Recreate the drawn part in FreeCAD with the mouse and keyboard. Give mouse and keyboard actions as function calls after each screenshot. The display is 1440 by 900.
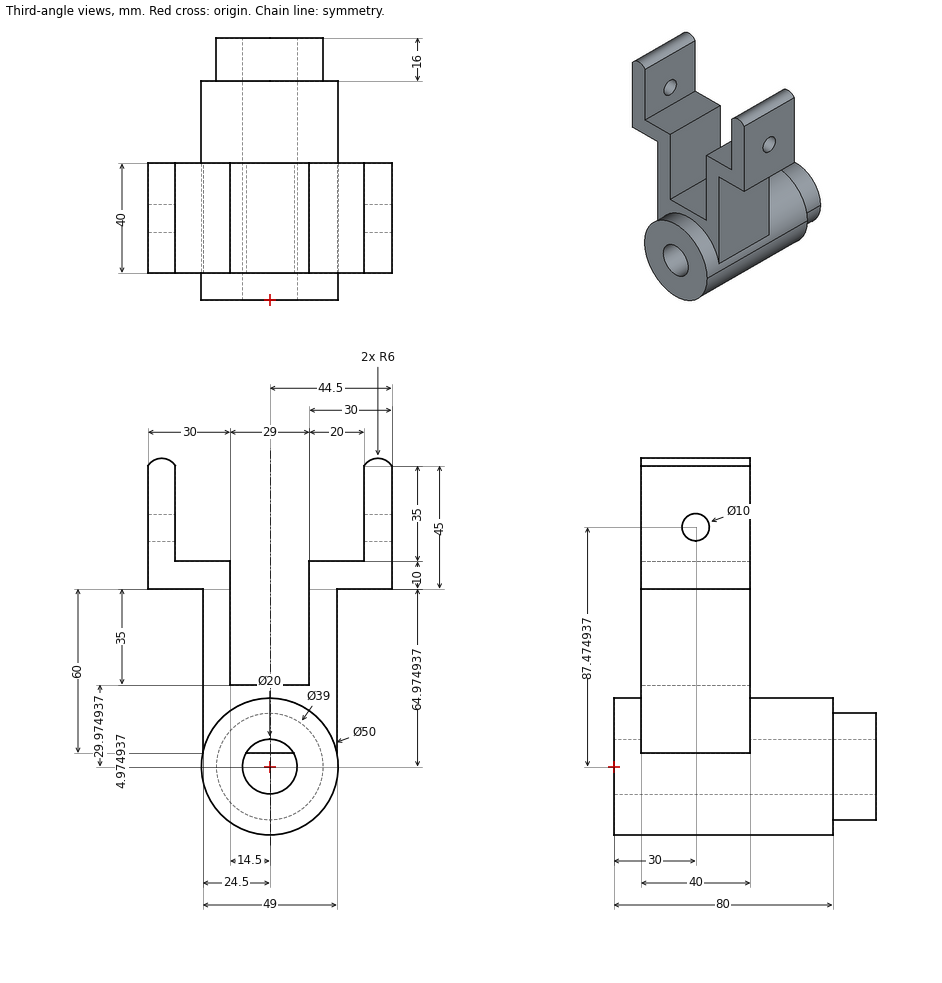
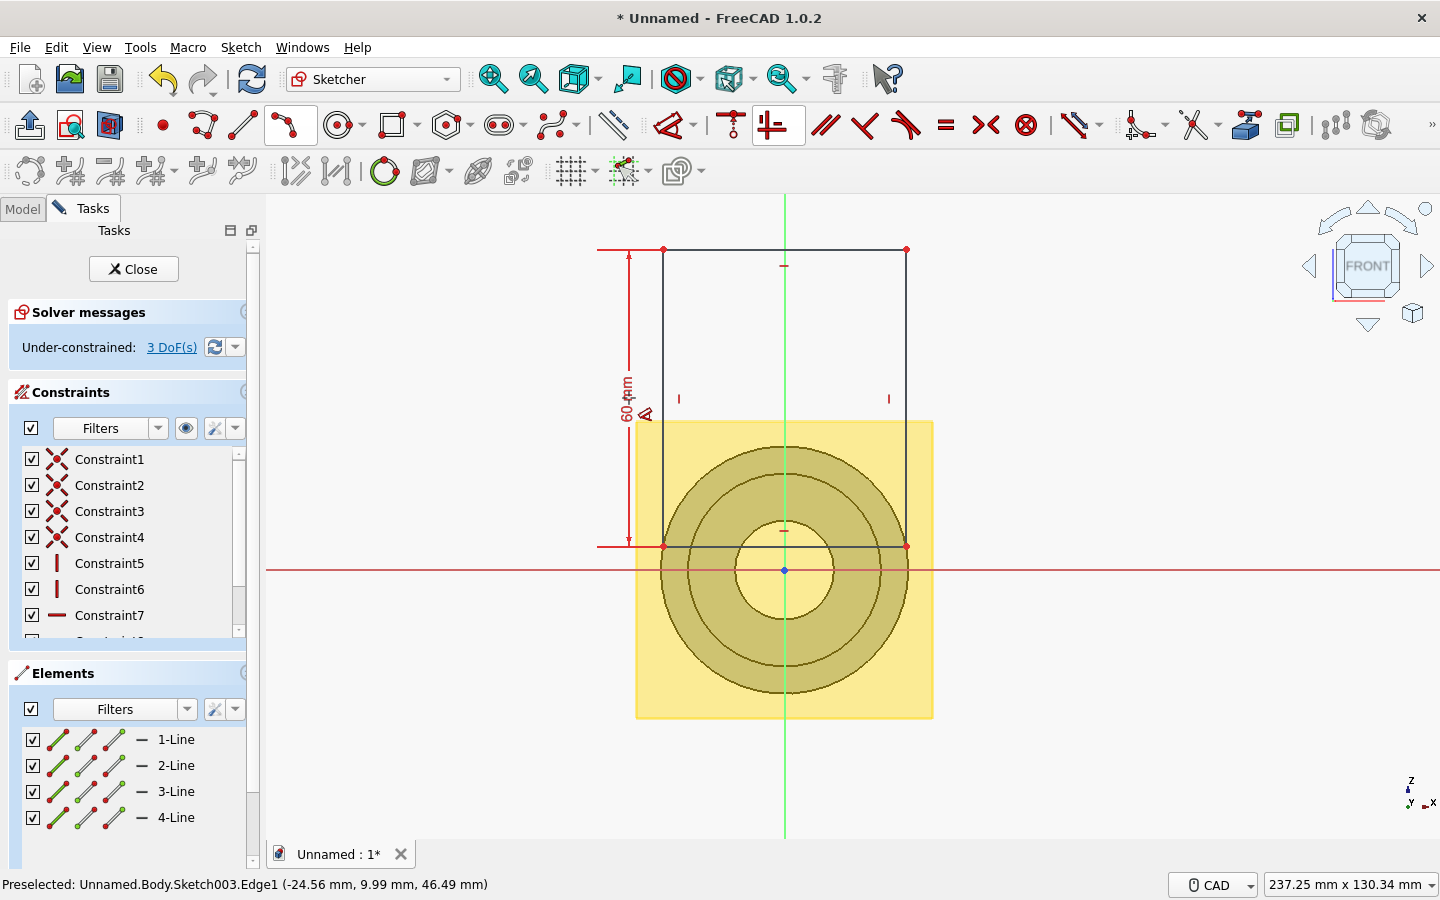
click(736, 547)
click(729, 513)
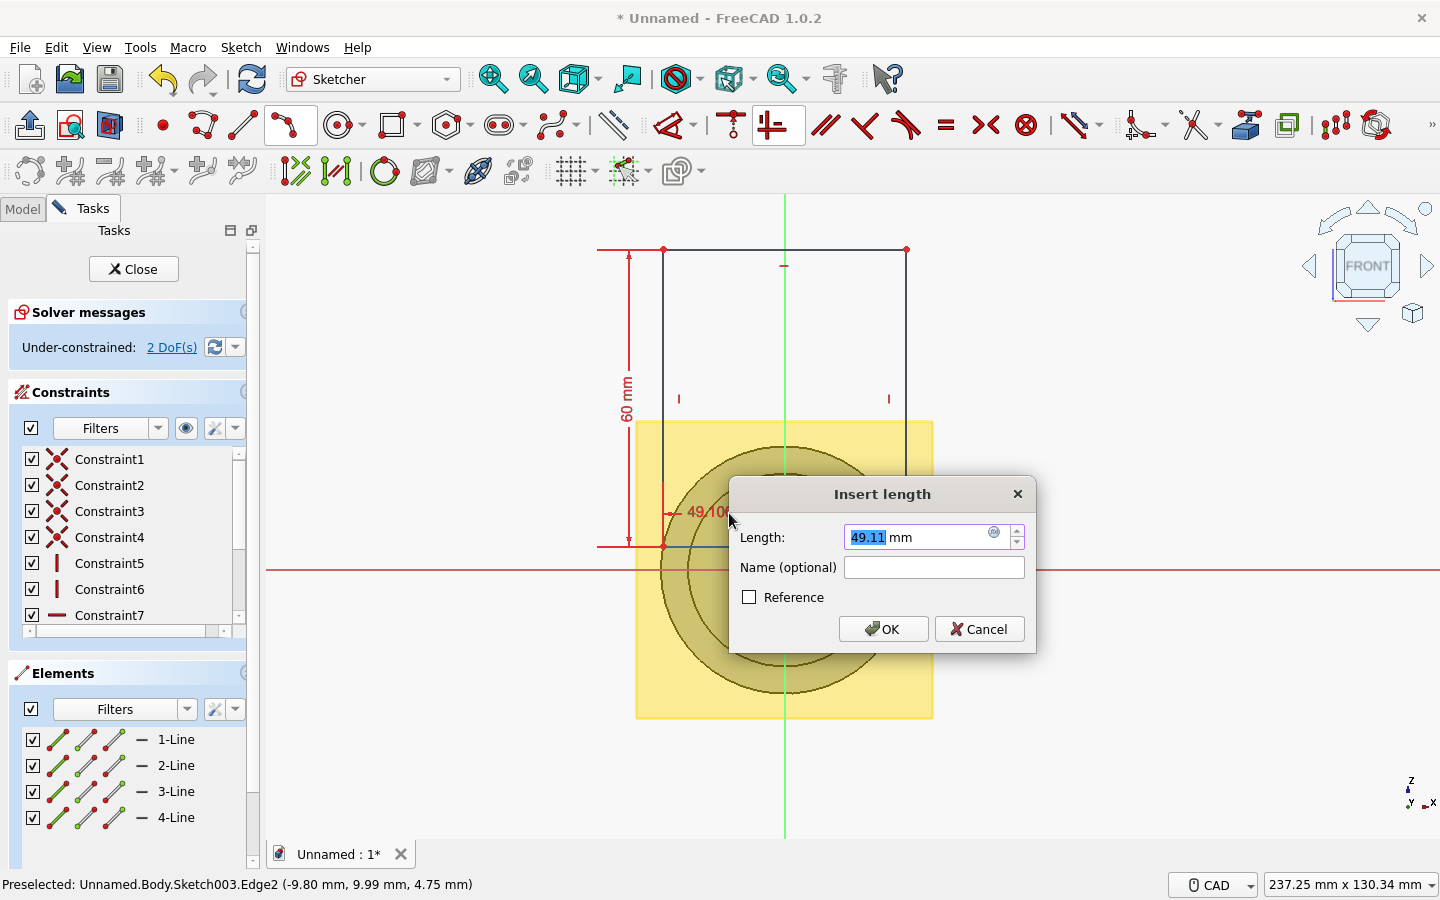
text(49)
key(Return)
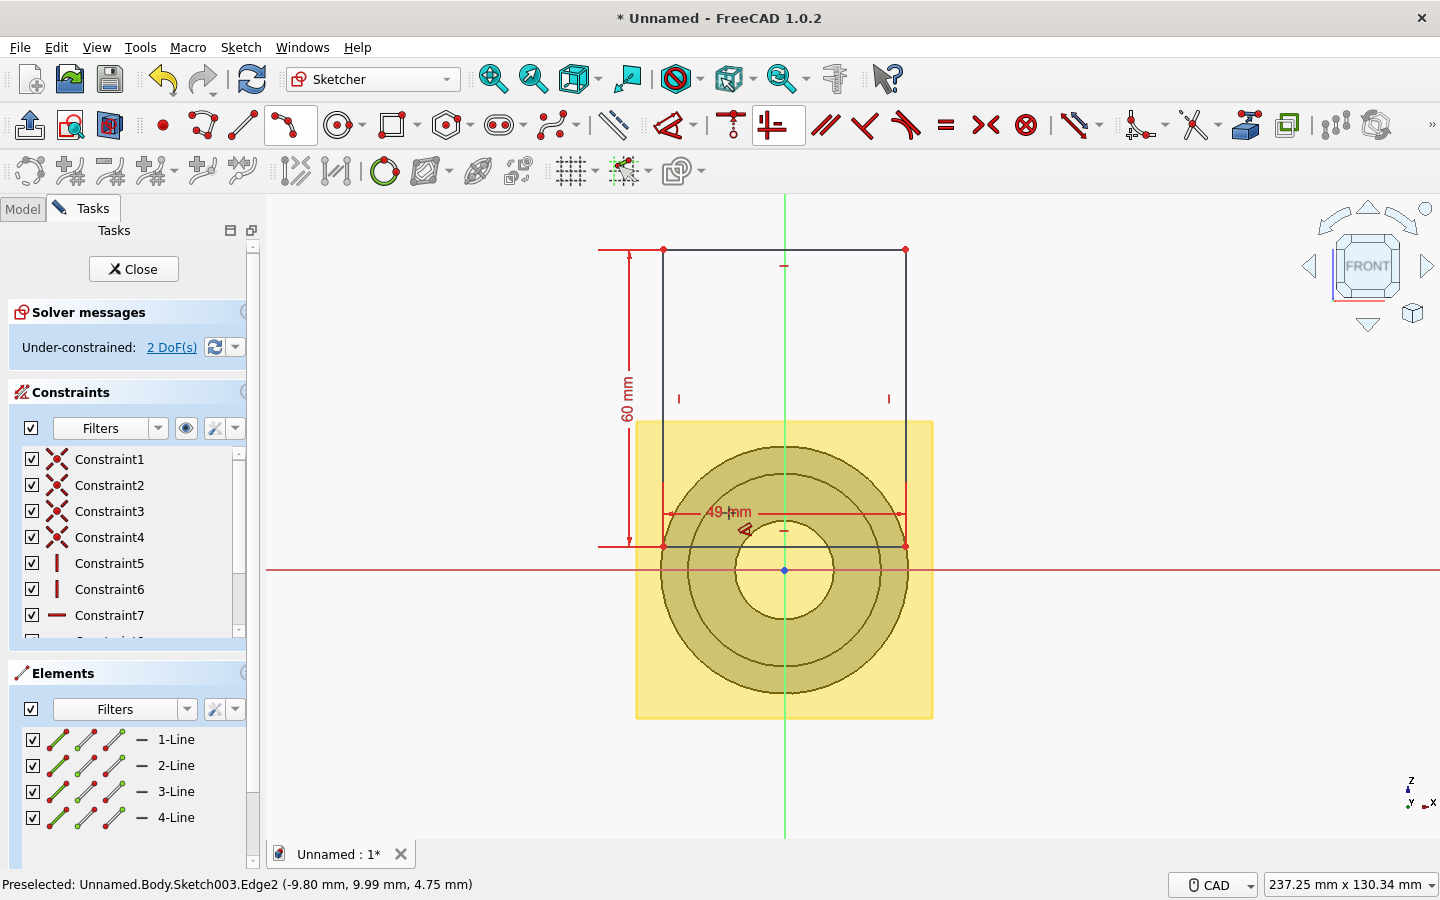
click(663, 250)
click(724, 604)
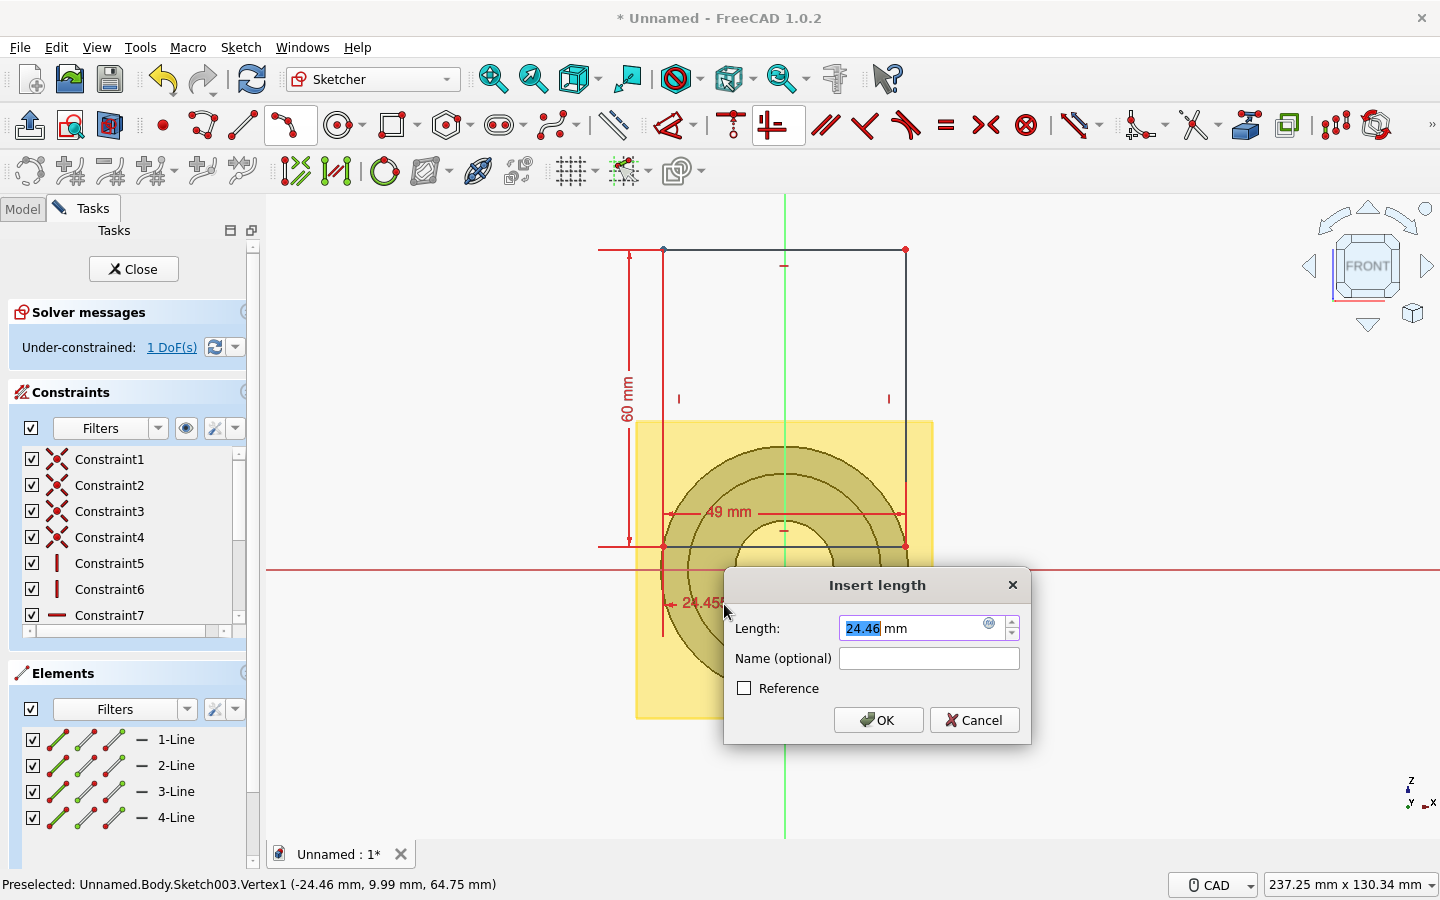
text(24.5)
key(Return)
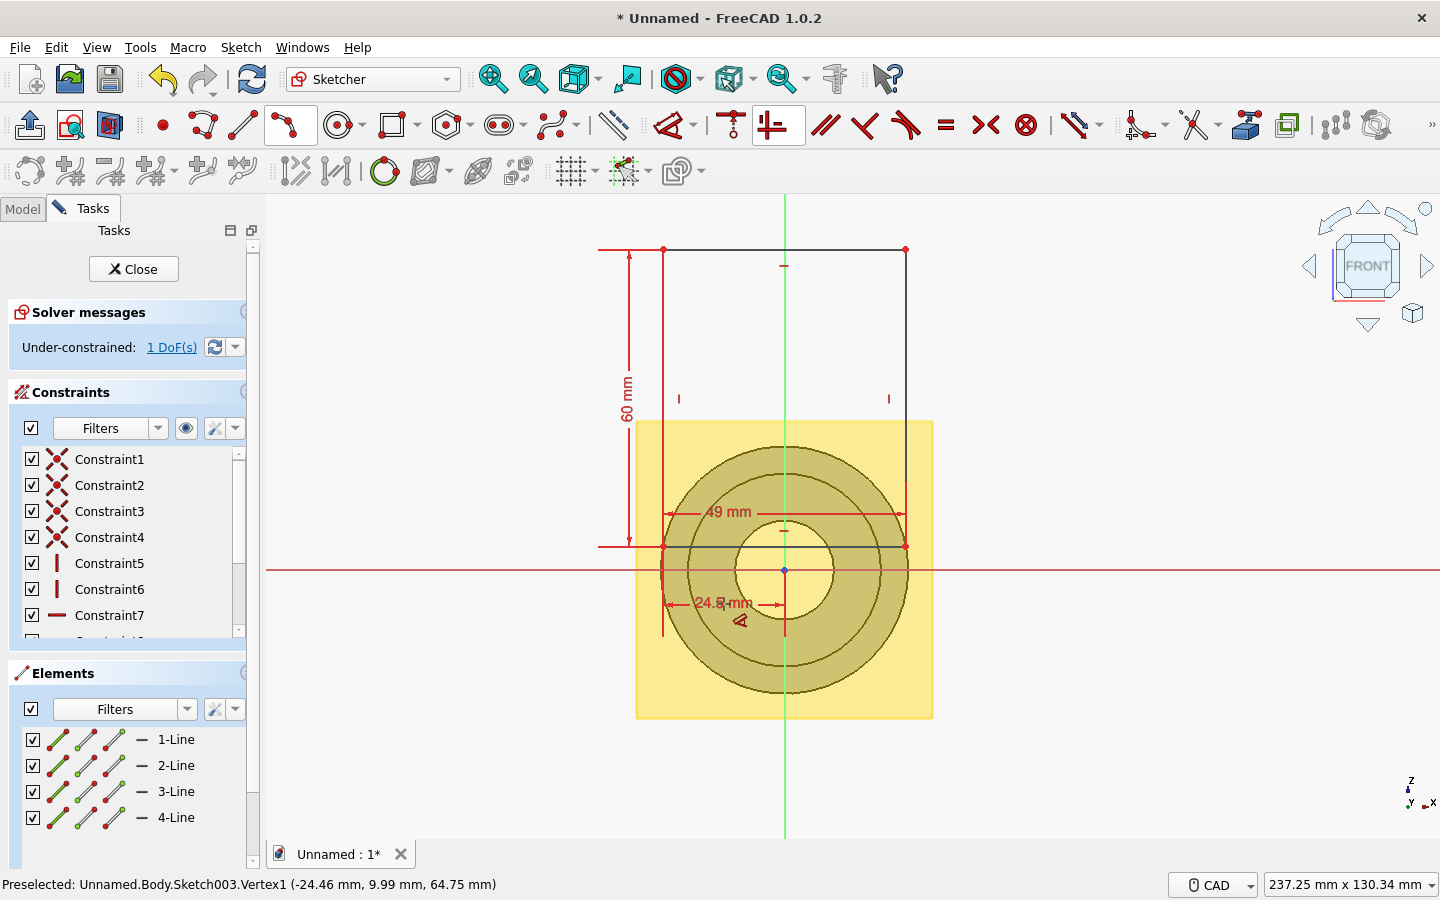
scroll(663, 547, up, 3)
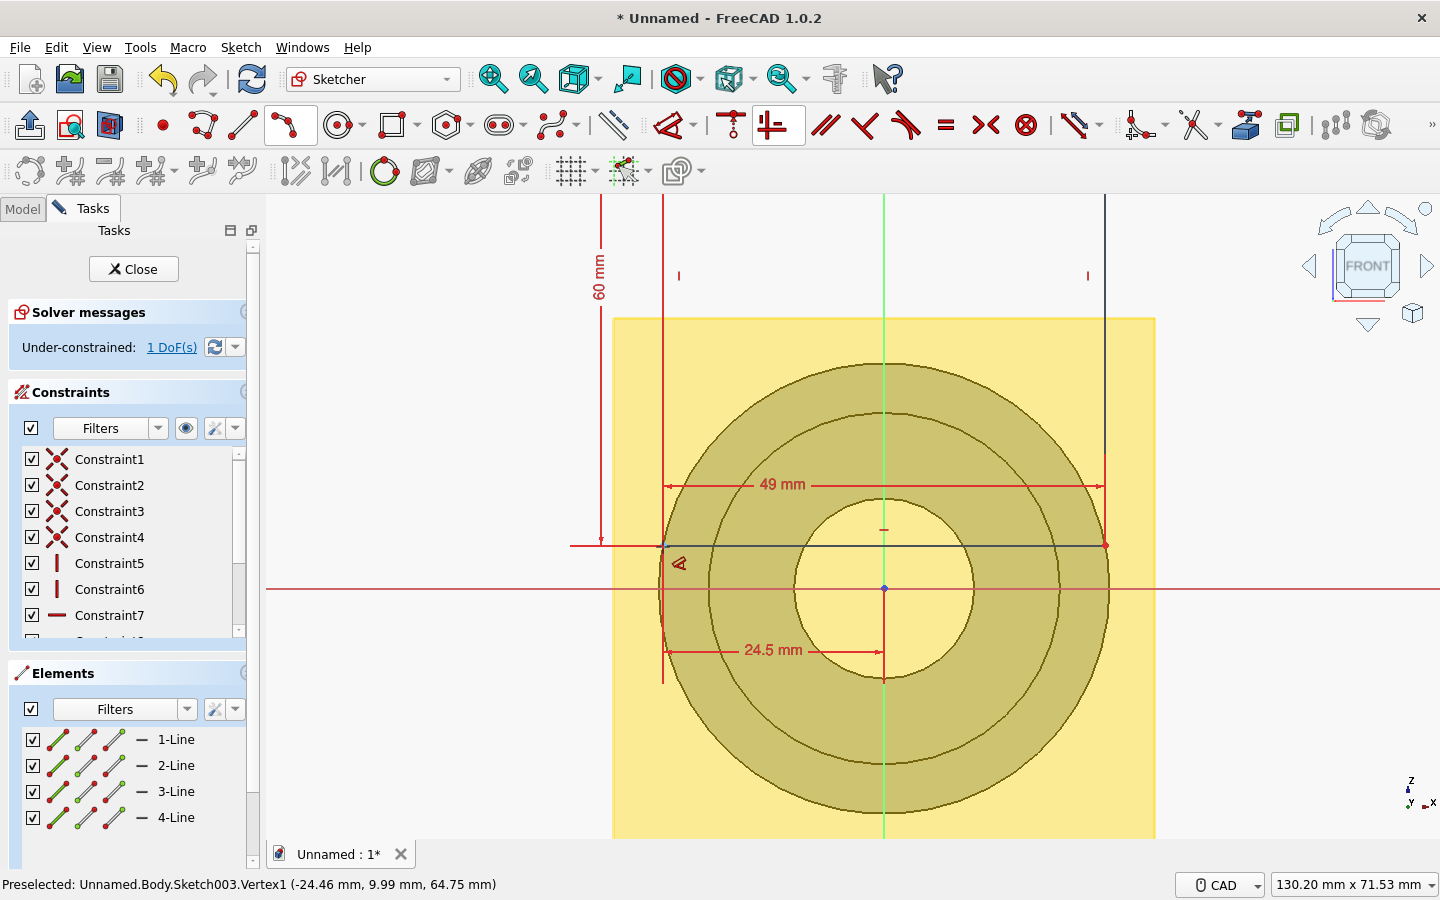
click(663, 546)
click(629, 567)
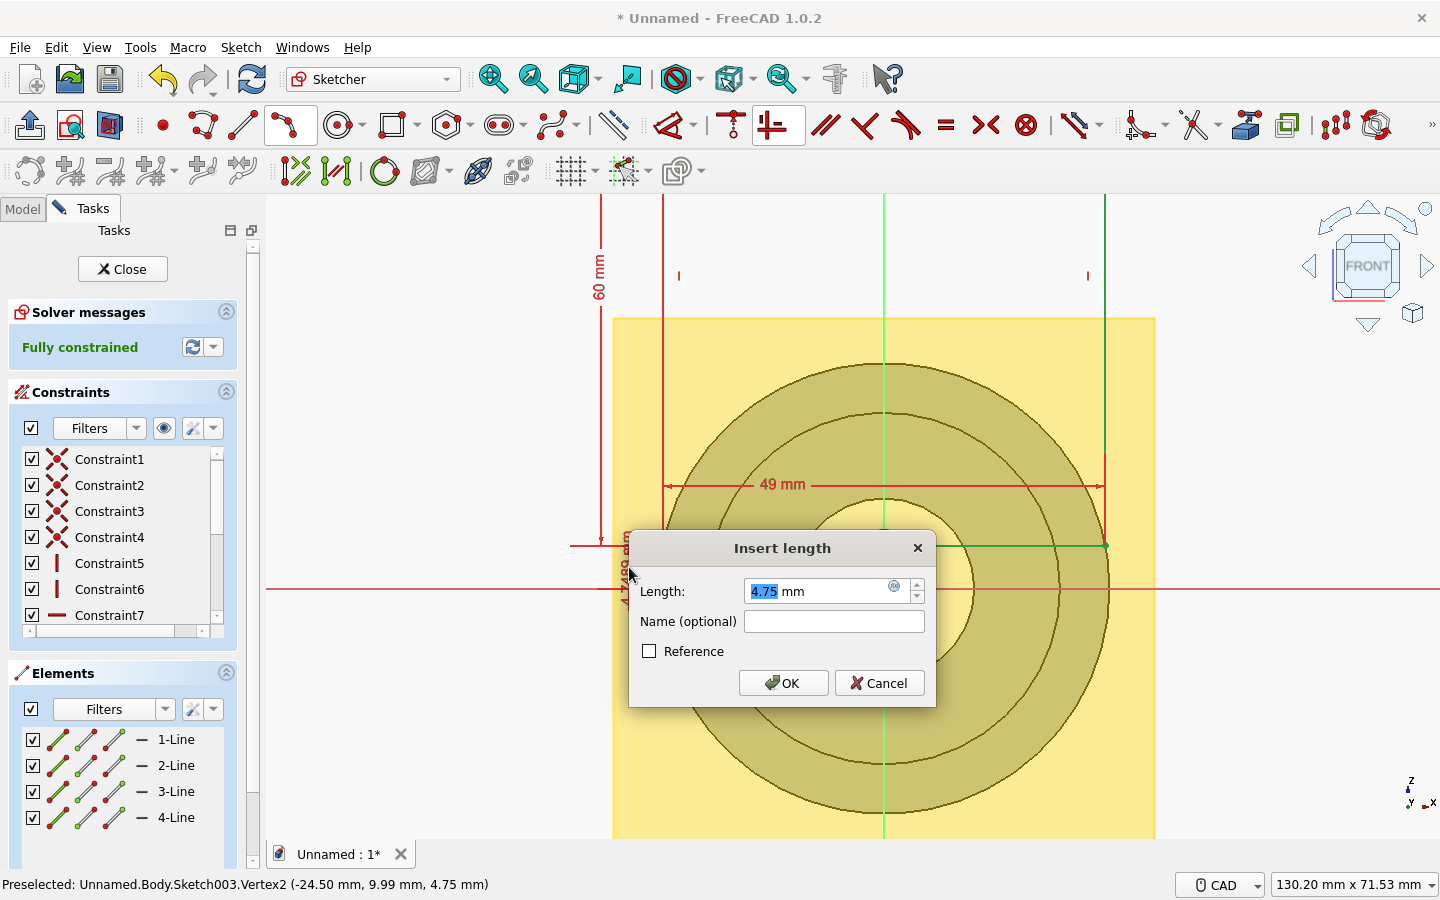
text(4.974937)
key(Return)
key(Escape)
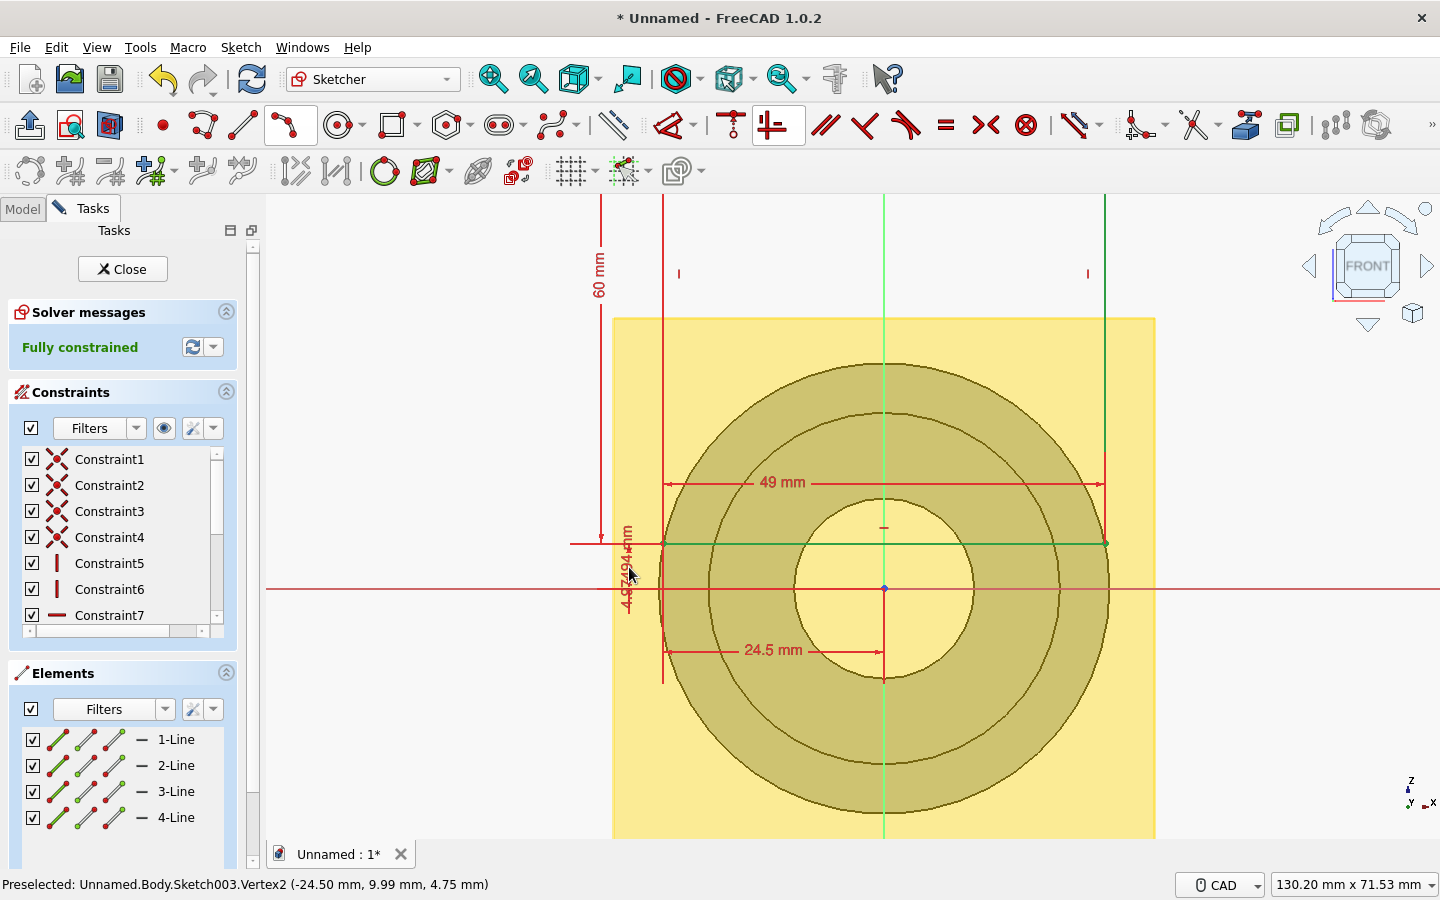
click(123, 269)